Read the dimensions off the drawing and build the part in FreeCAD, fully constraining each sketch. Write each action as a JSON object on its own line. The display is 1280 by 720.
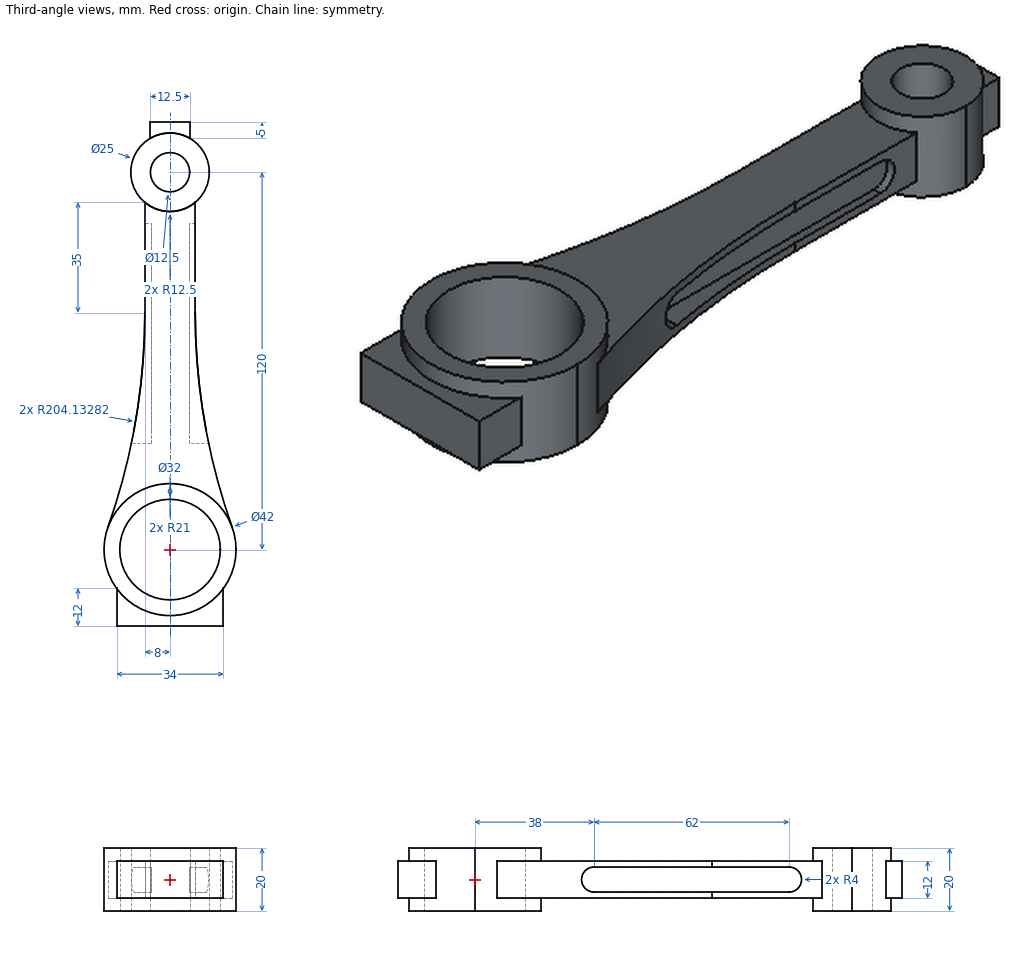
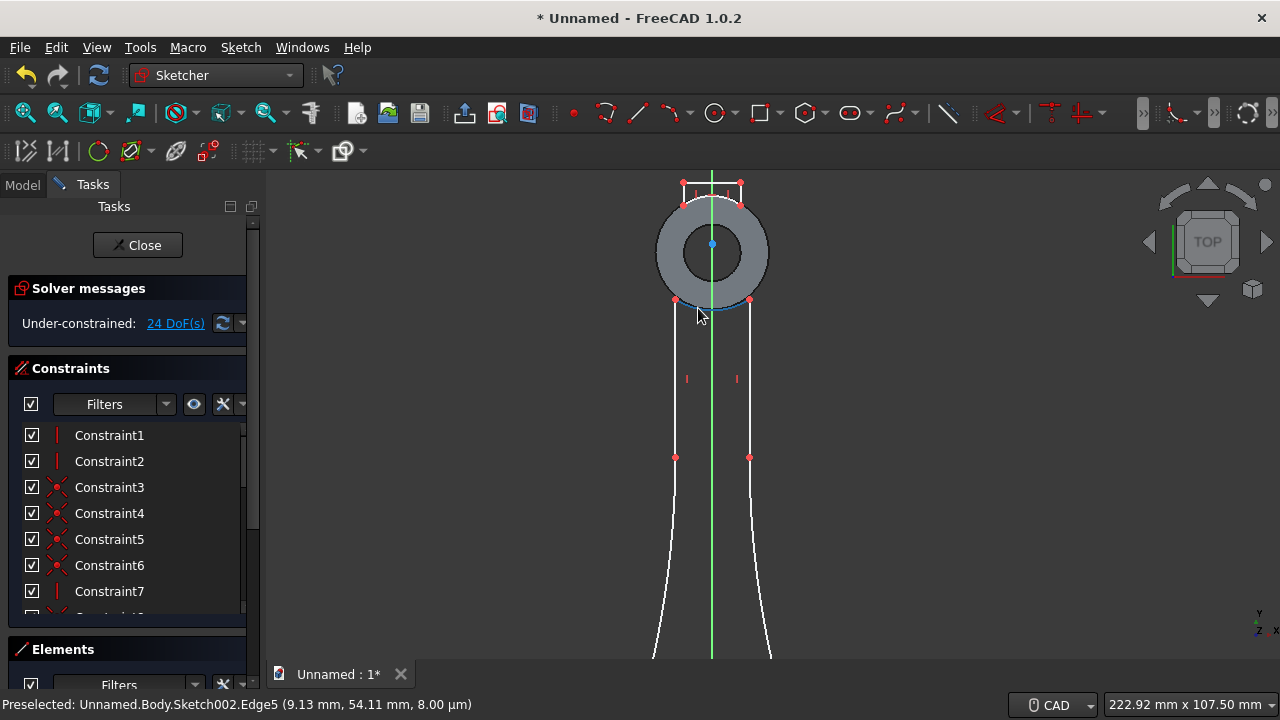
{"action": "left_click", "coordinate": [697, 308]}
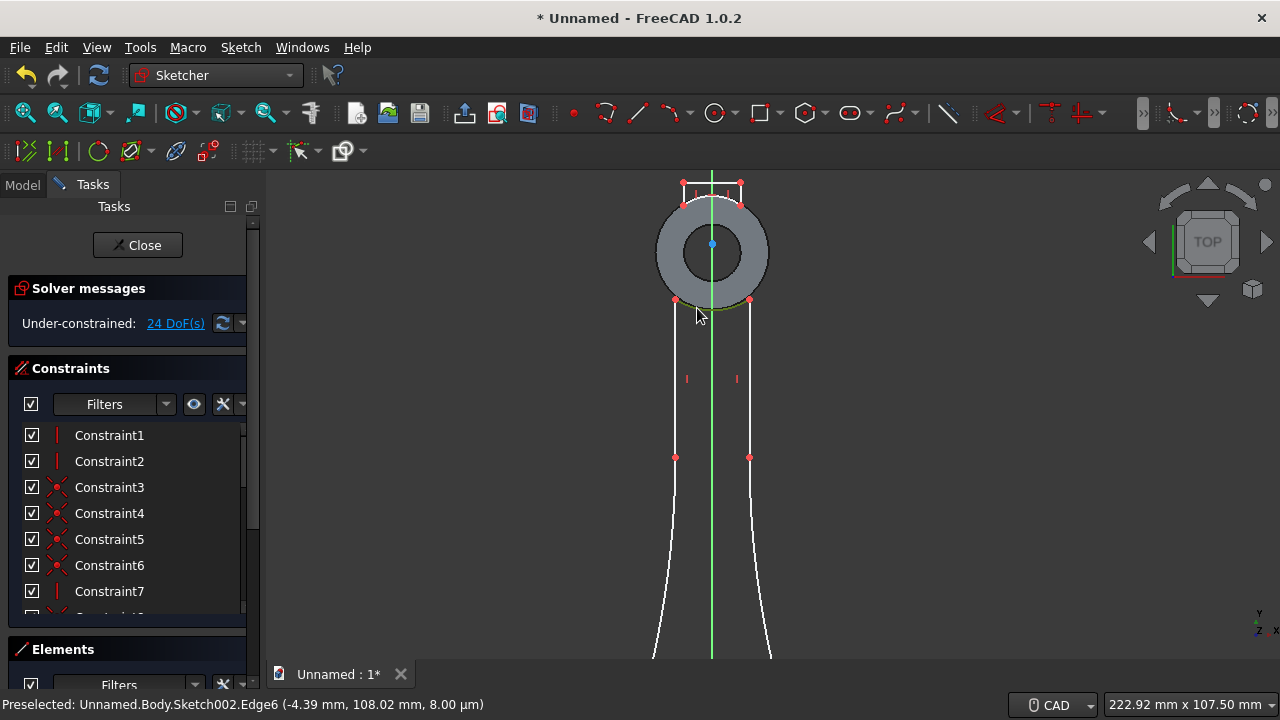
{"action": "scroll", "coordinate": [730, 199], "scroll_direction": "up", "scroll_amount": 2}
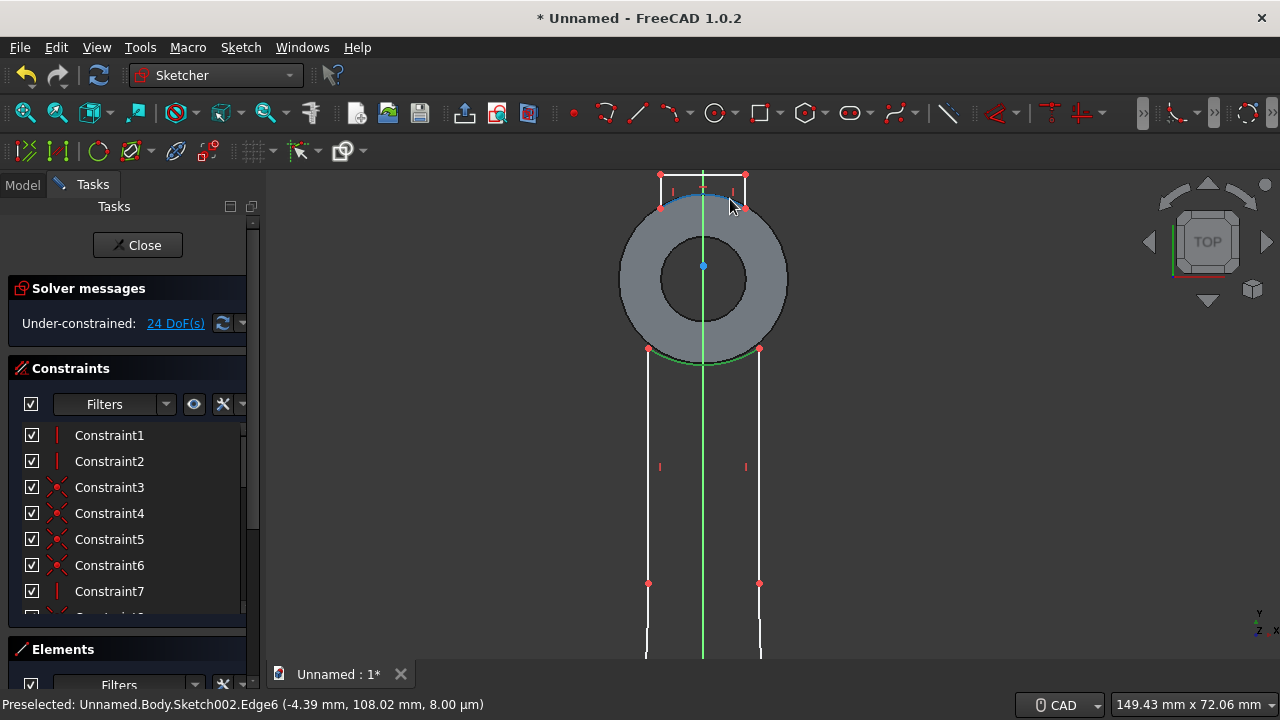
{"action": "left_click", "coordinate": [730, 199]}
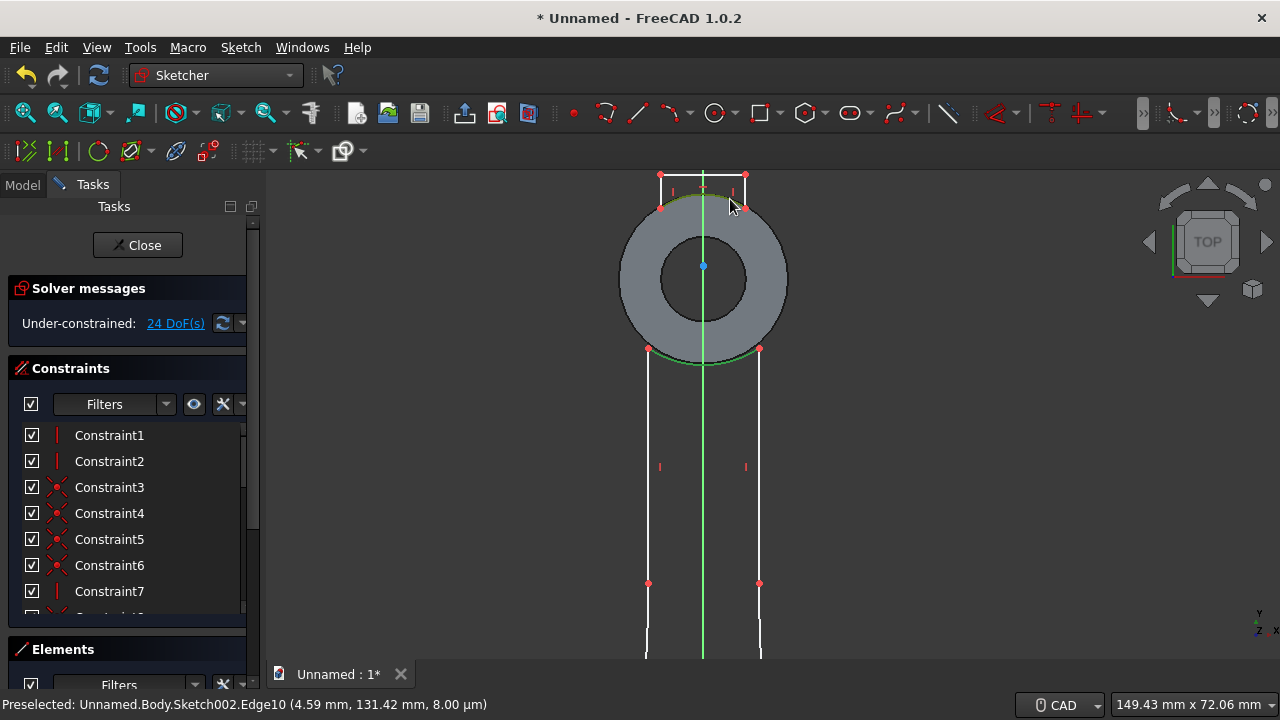
{"action": "key", "text": "c"}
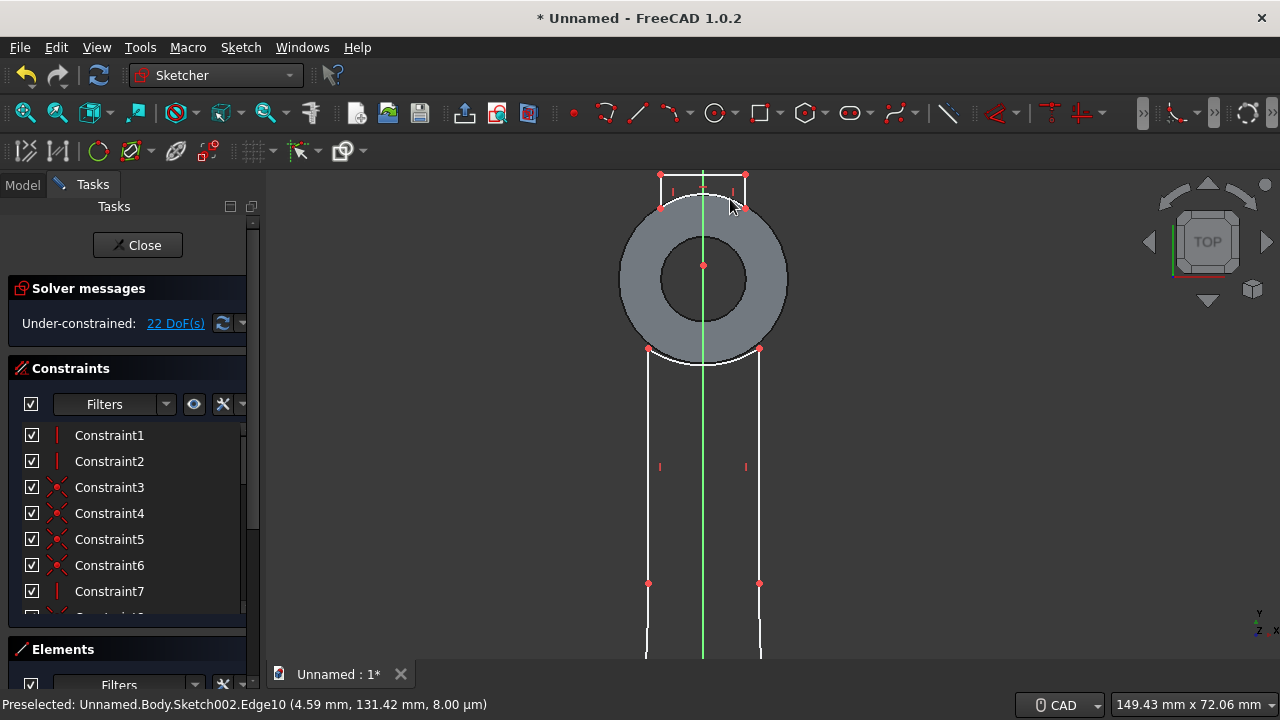
{"action": "scroll", "coordinate": [705, 285], "scroll_direction": "down", "scroll_amount": 6}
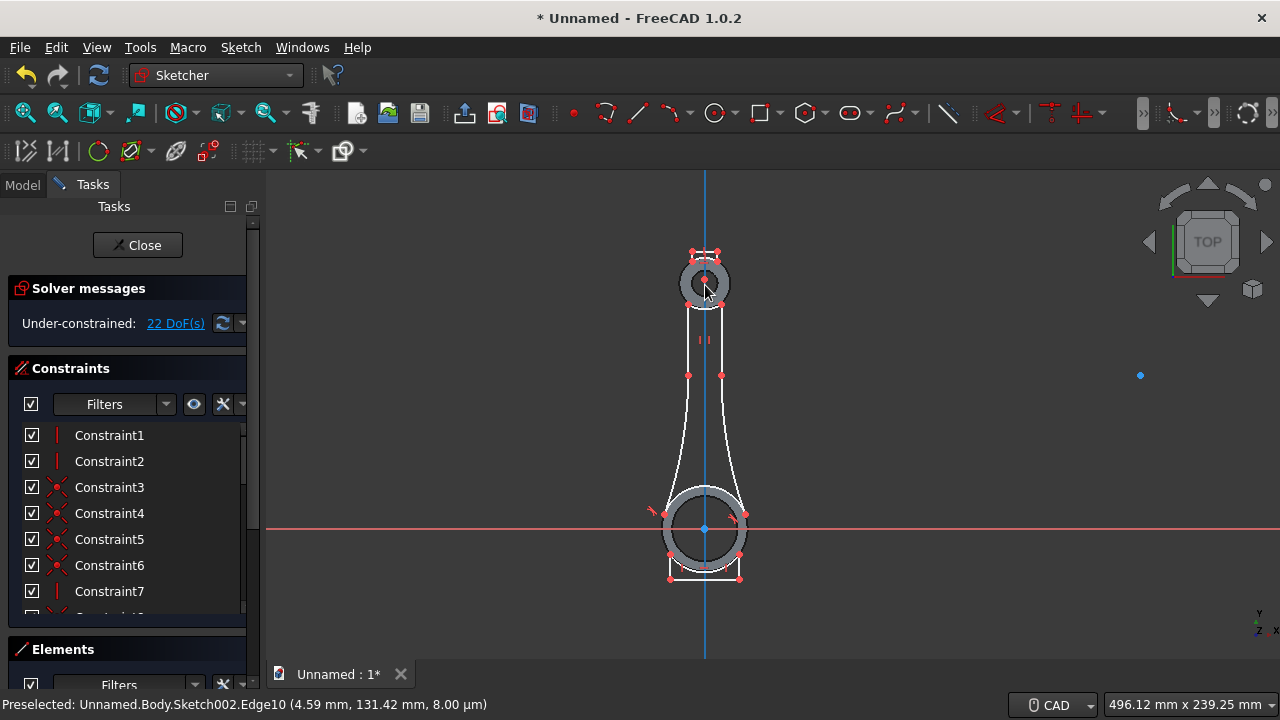
{"action": "left_click", "coordinate": [725, 491]}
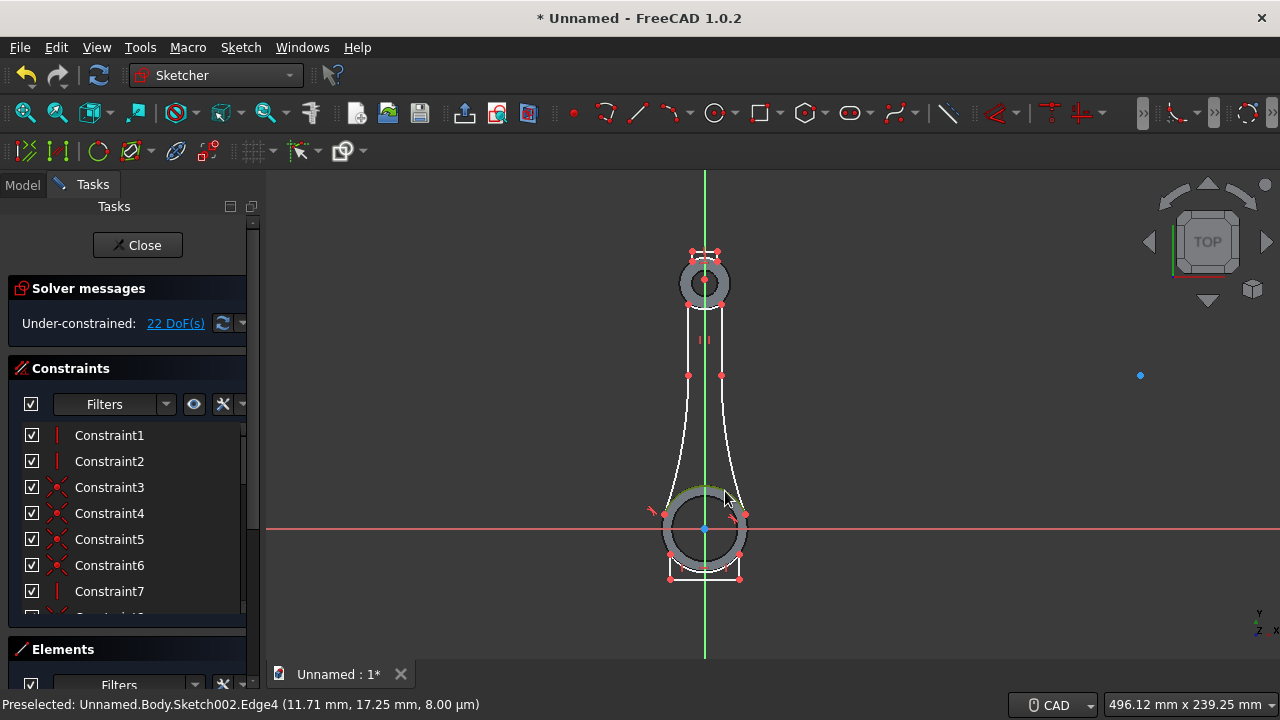
{"action": "scroll", "coordinate": [689, 569], "scroll_direction": "up", "scroll_amount": 2}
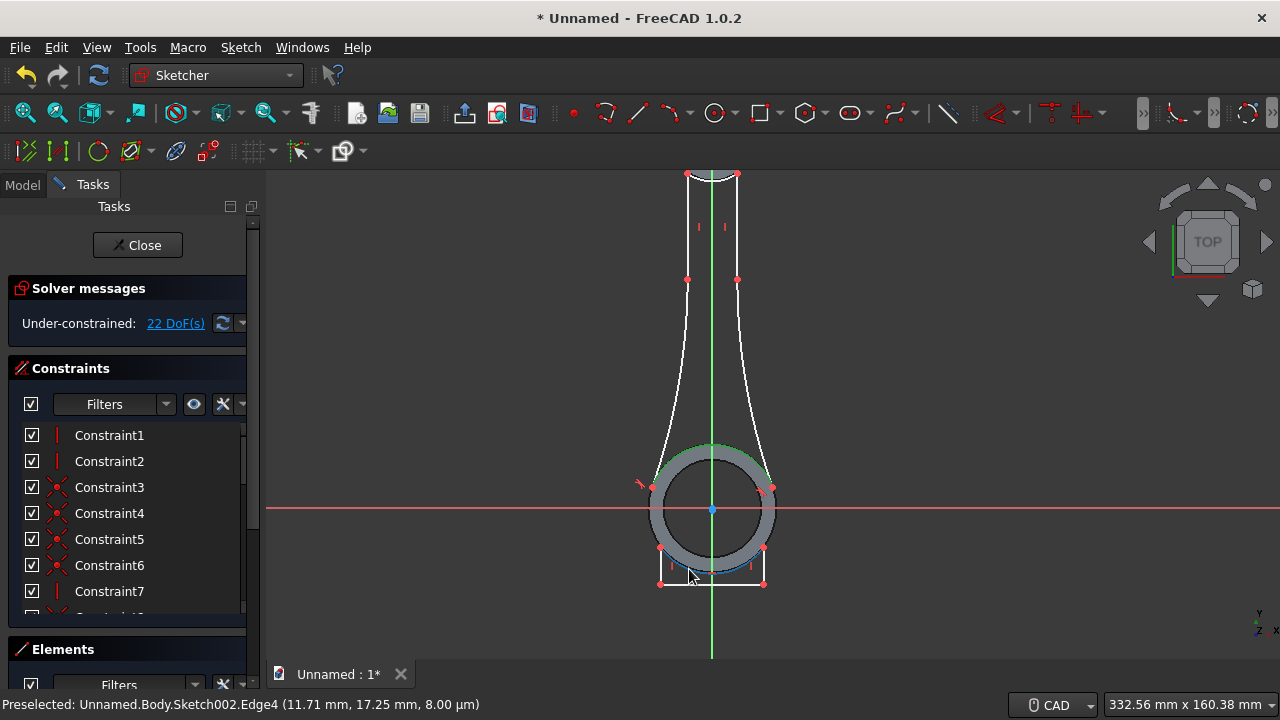
{"action": "left_click", "coordinate": [689, 569]}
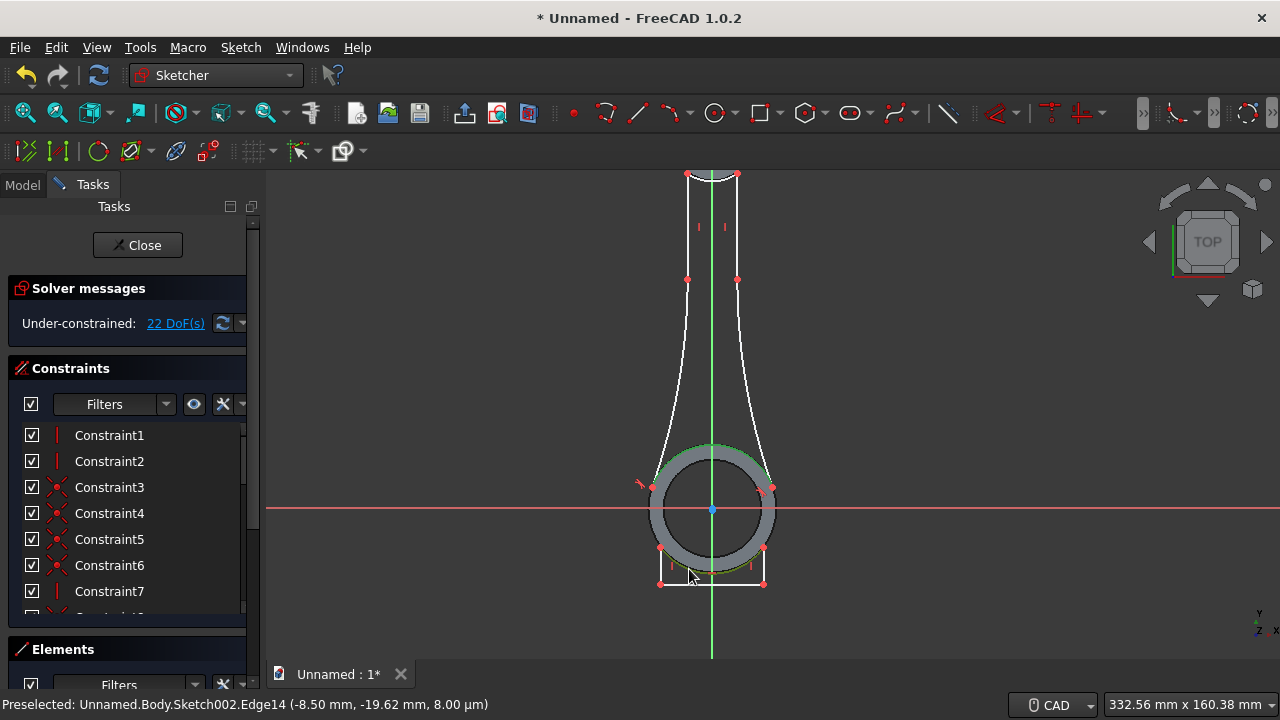
{"action": "left_click", "coordinate": [1050, 114]}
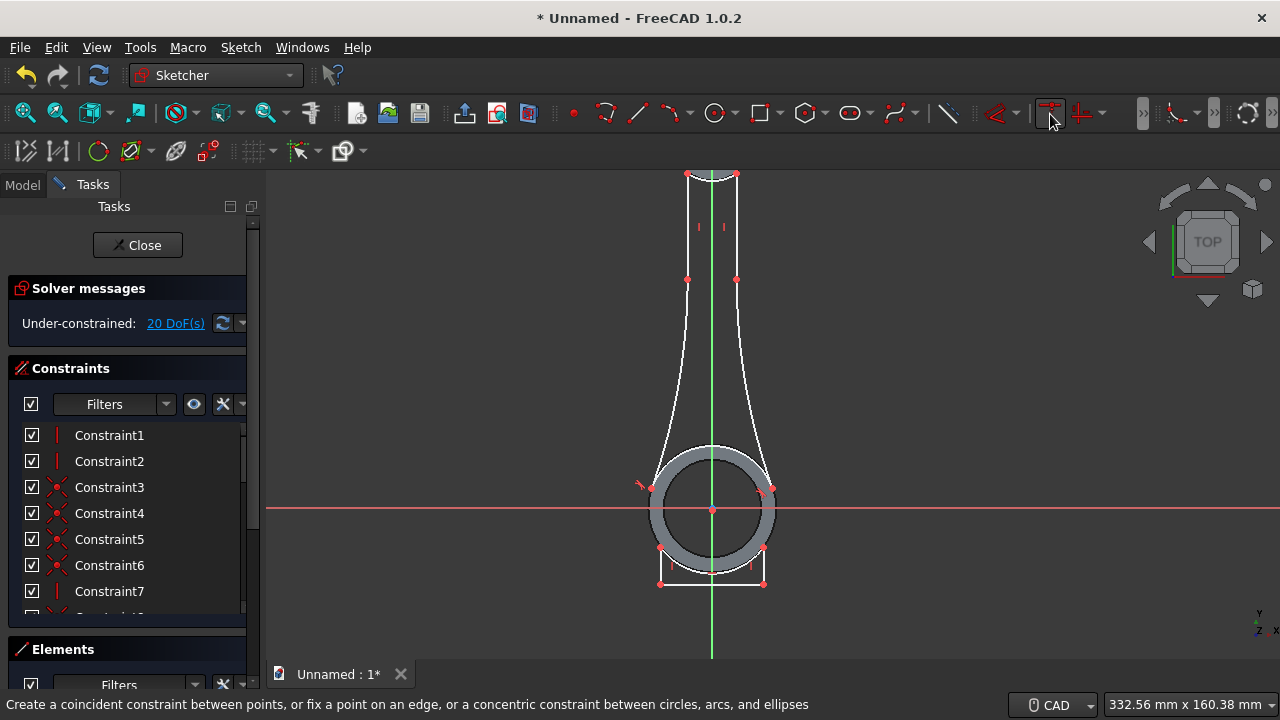
{"action": "scroll", "coordinate": [712, 509], "scroll_direction": "up", "scroll_amount": 2}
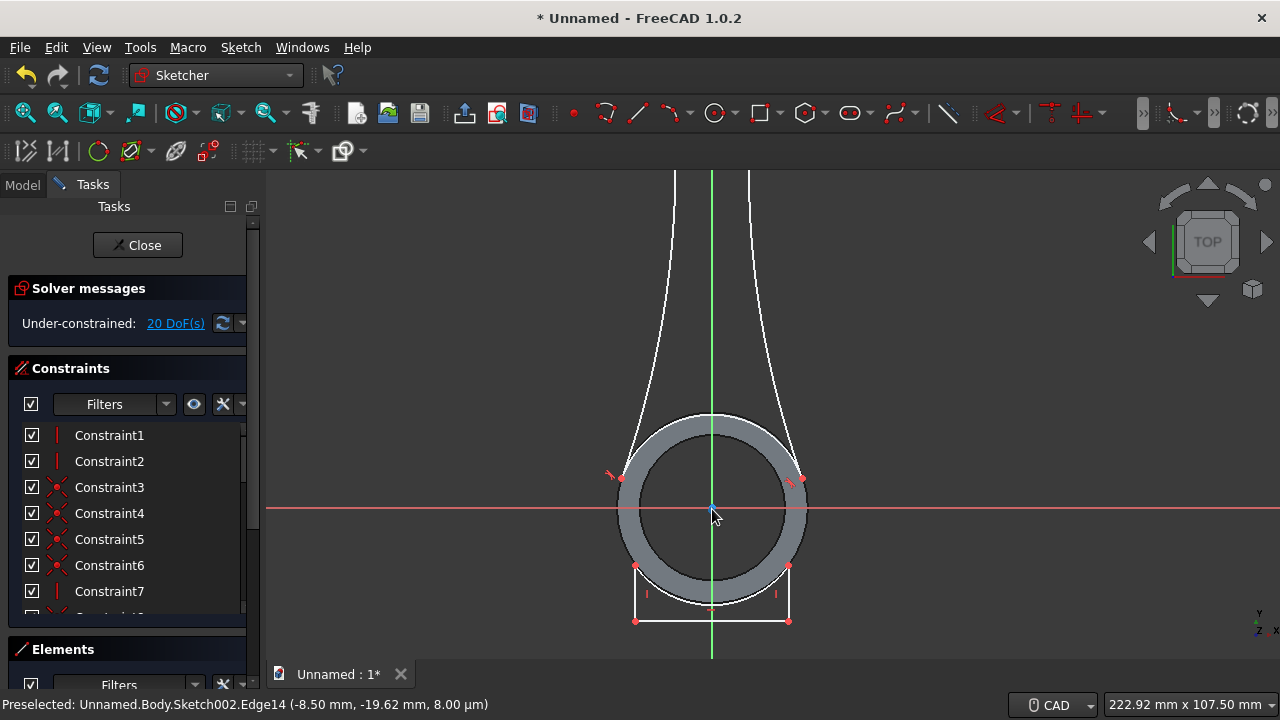
{"action": "left_click_drag", "start_coordinate": [702, 498], "coordinate": [722, 520]}